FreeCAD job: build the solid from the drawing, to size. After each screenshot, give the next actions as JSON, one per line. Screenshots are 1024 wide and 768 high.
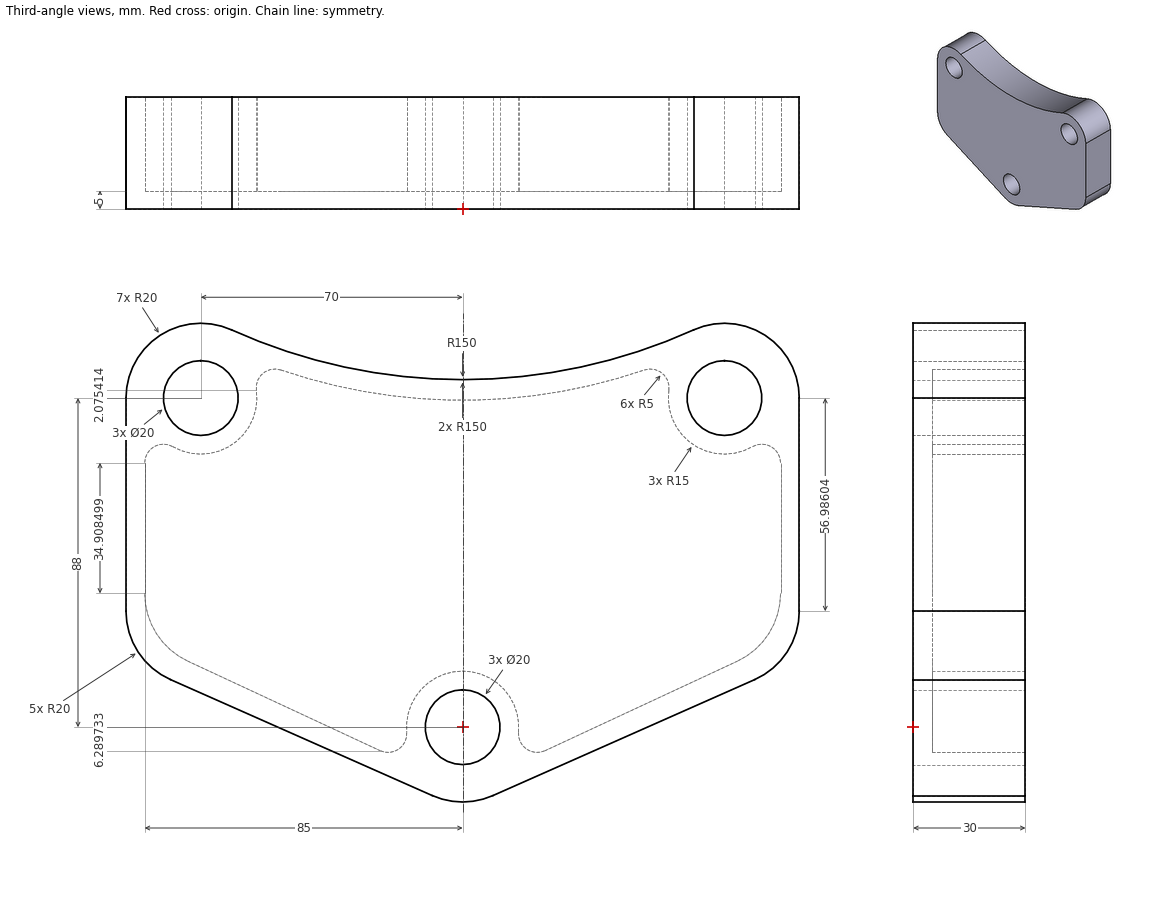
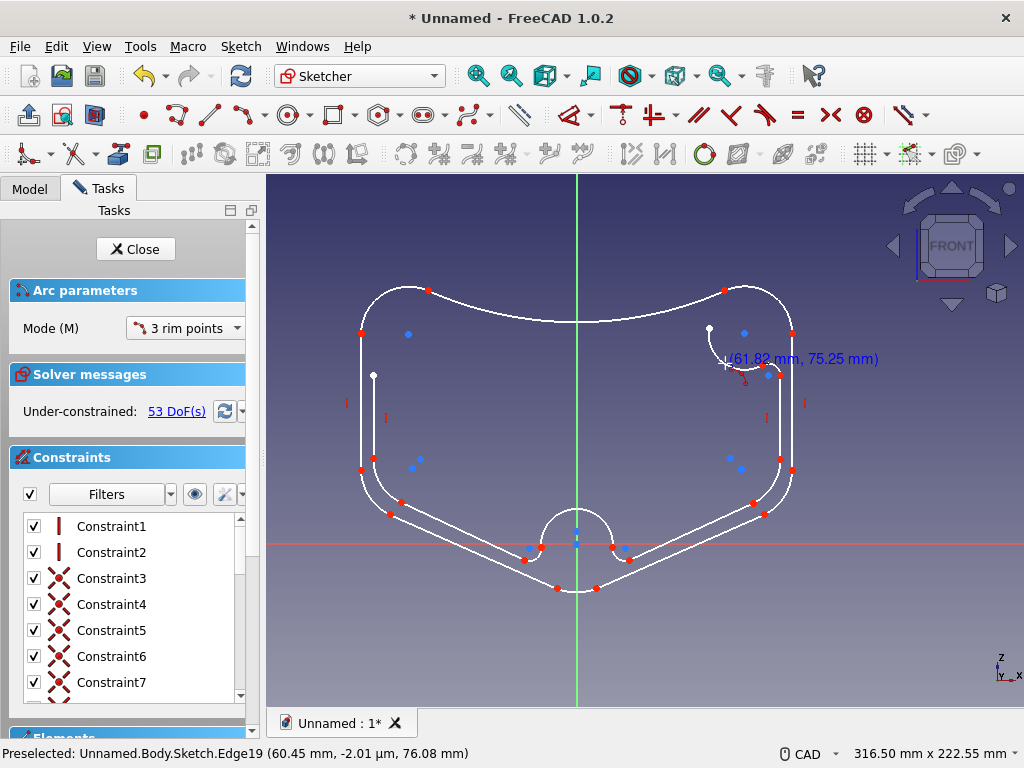
{"action": "left_click", "coordinate": [709, 329]}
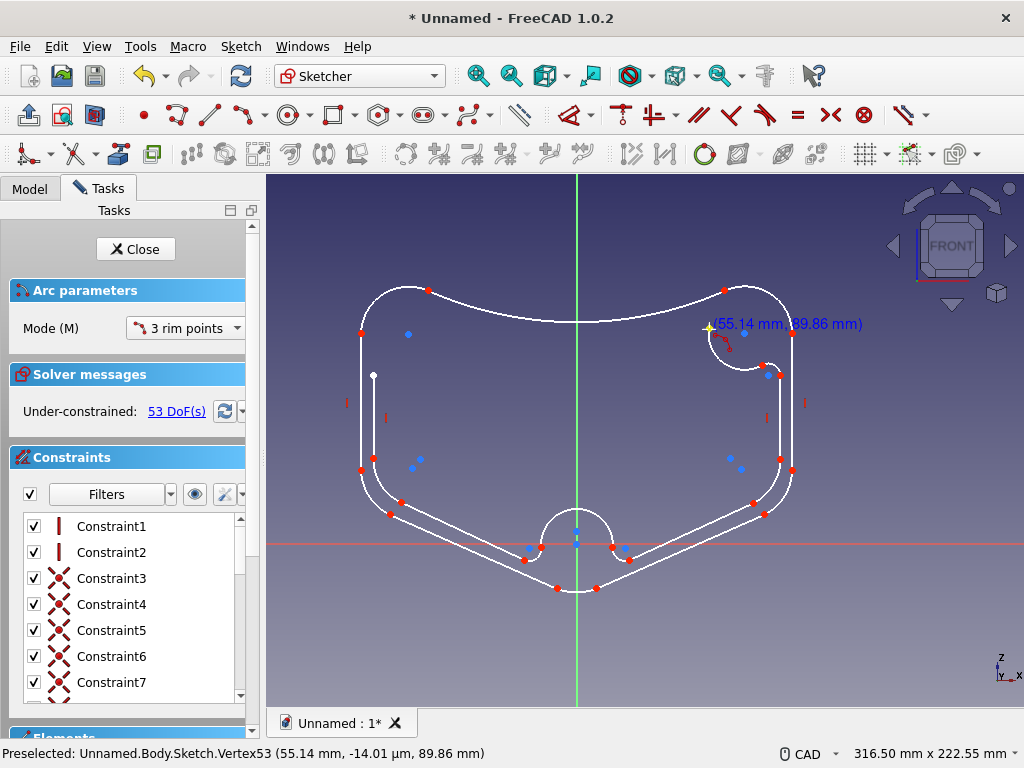
{"action": "scroll", "coordinate": [693, 316], "scroll_direction": "up", "scroll_amount": 2}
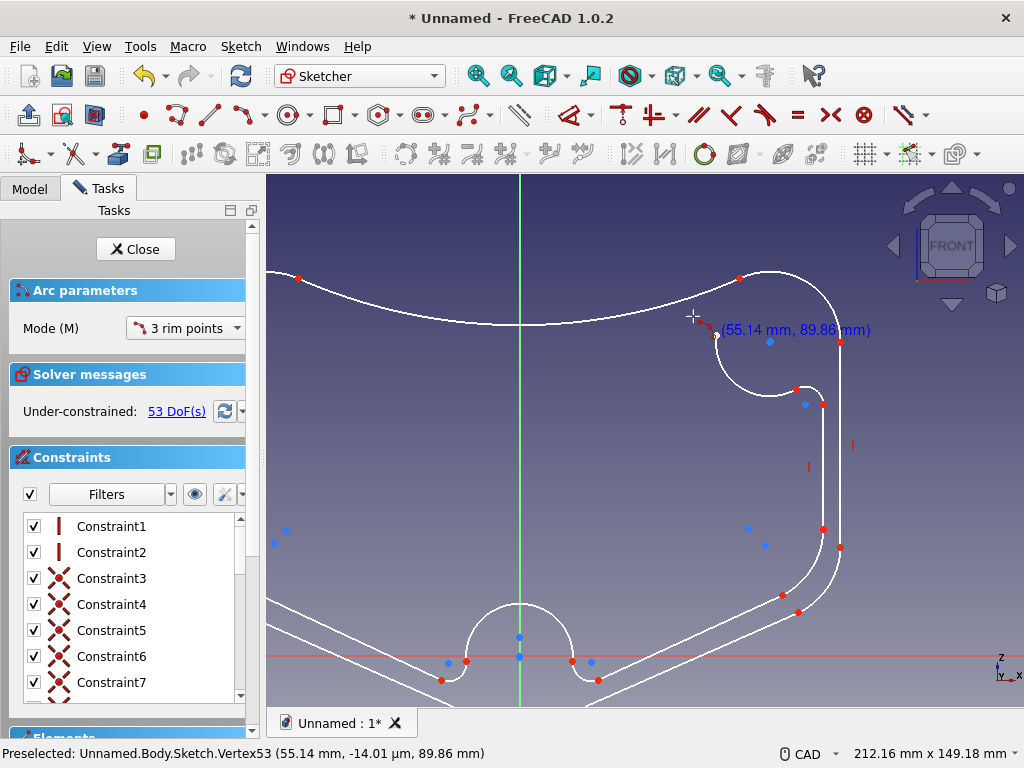
{"action": "left_click", "coordinate": [693, 315]}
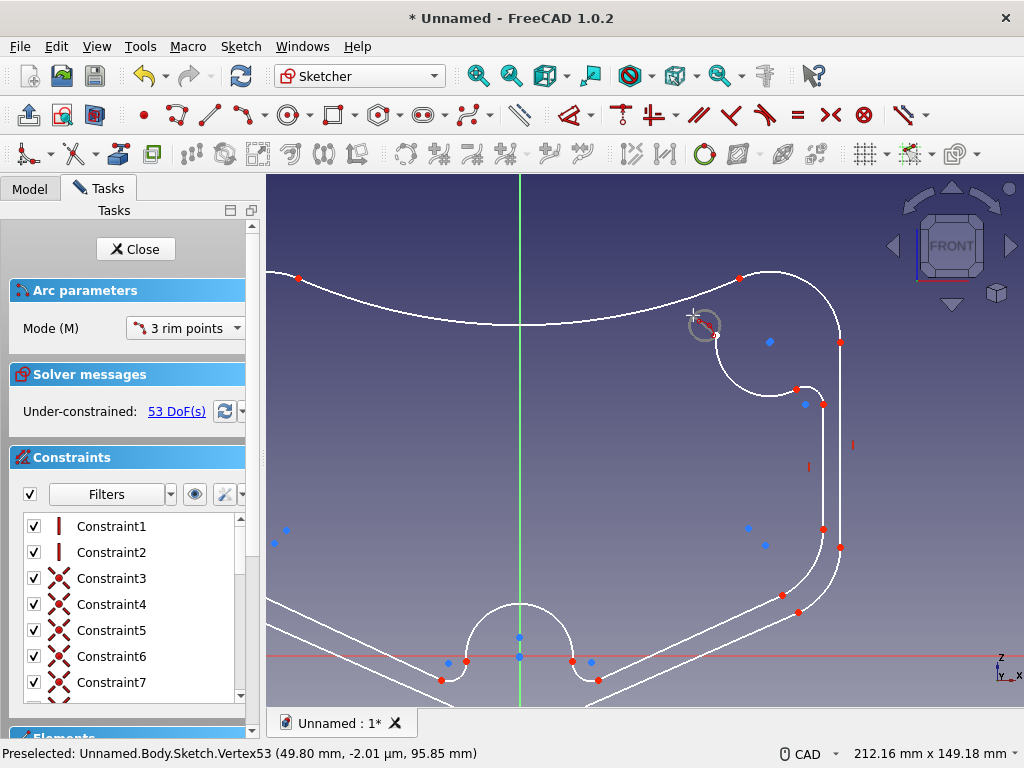
{"action": "scroll", "coordinate": [710, 318], "scroll_direction": "up", "scroll_amount": 4}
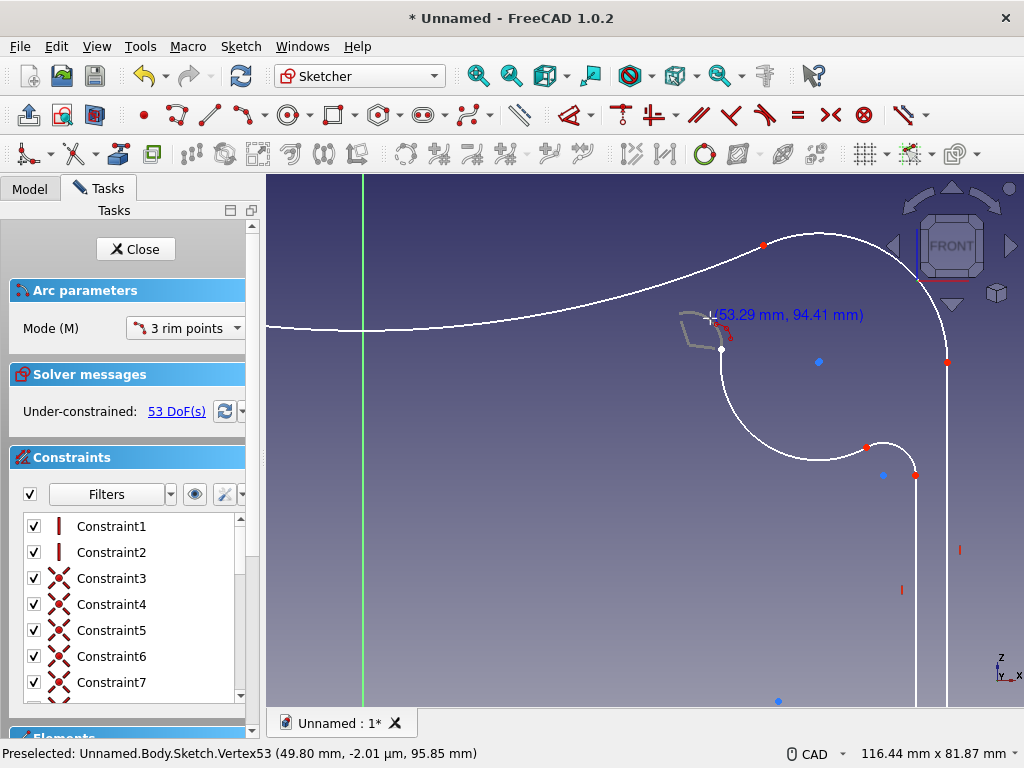
{"action": "left_click", "coordinate": [710, 318]}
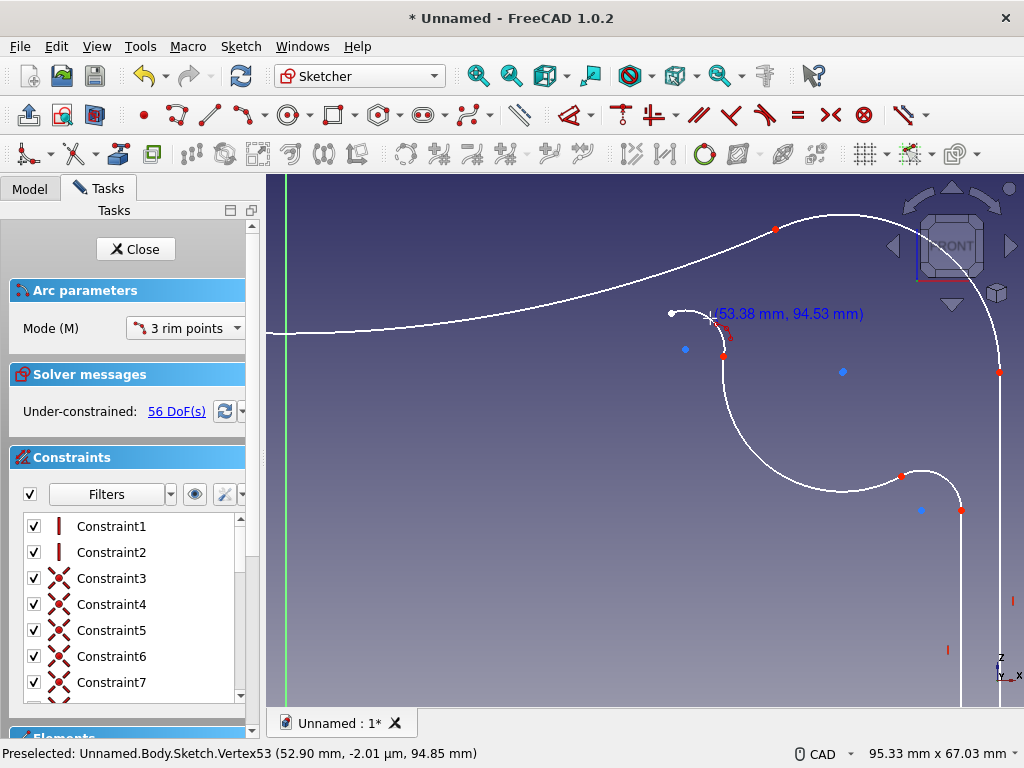
{"action": "left_click", "coordinate": [671, 313]}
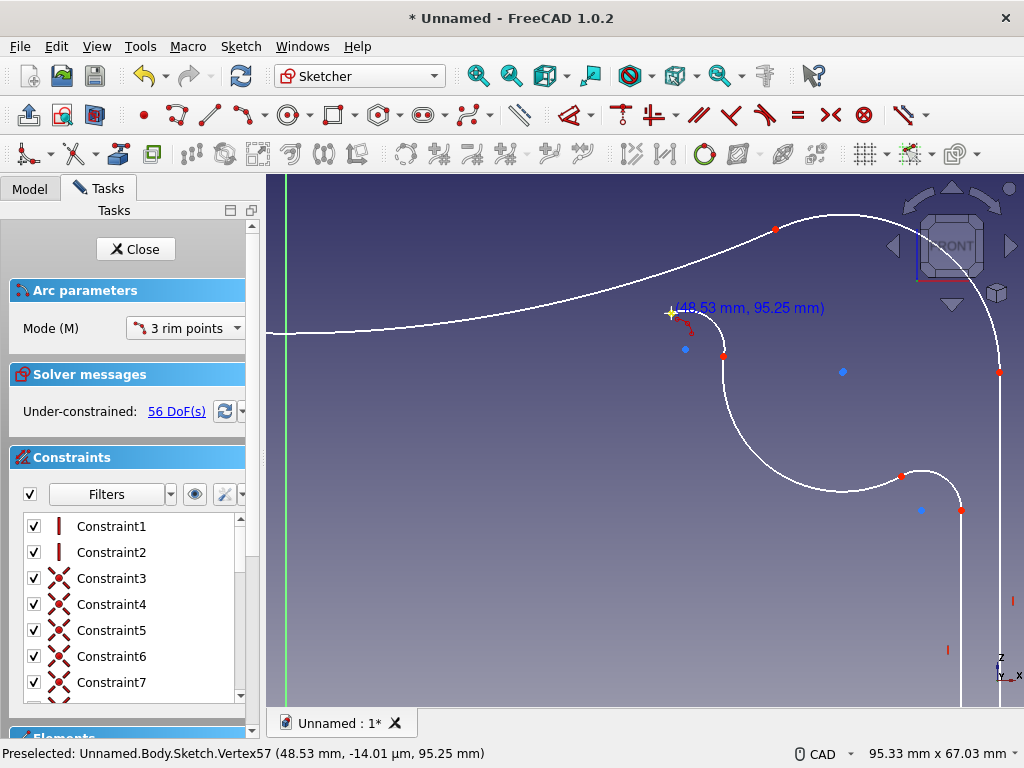
{"action": "scroll", "coordinate": [702, 317], "scroll_direction": "down", "scroll_amount": 6}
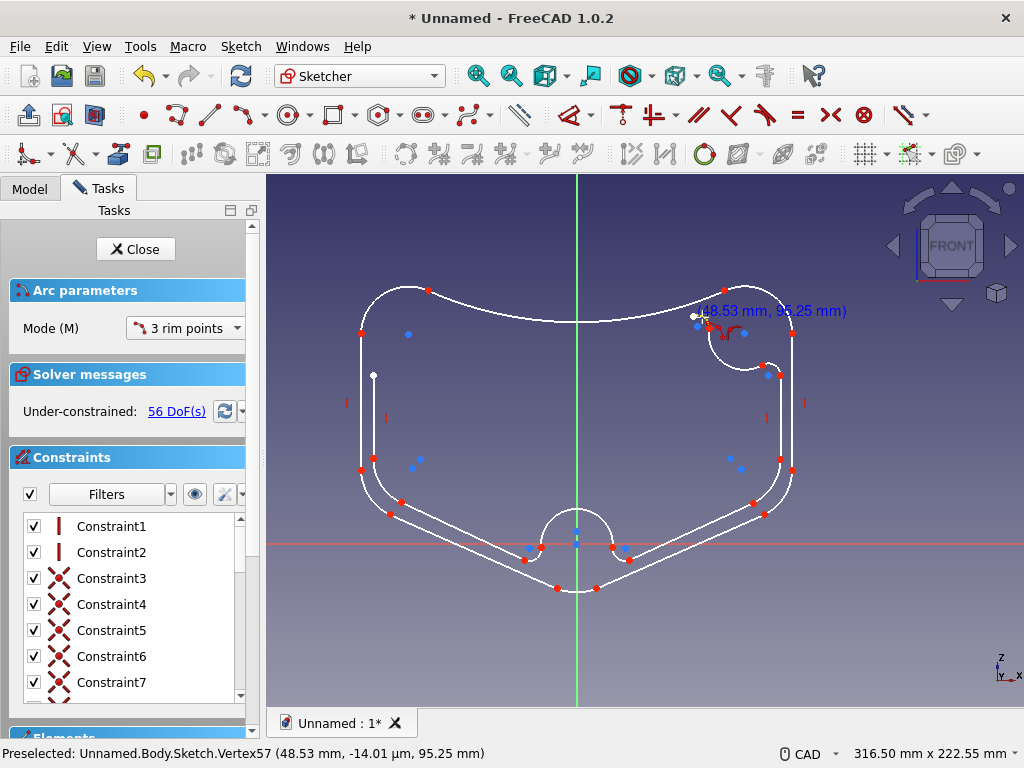
{"action": "scroll", "coordinate": [461, 315], "scroll_direction": "up", "scroll_amount": 2}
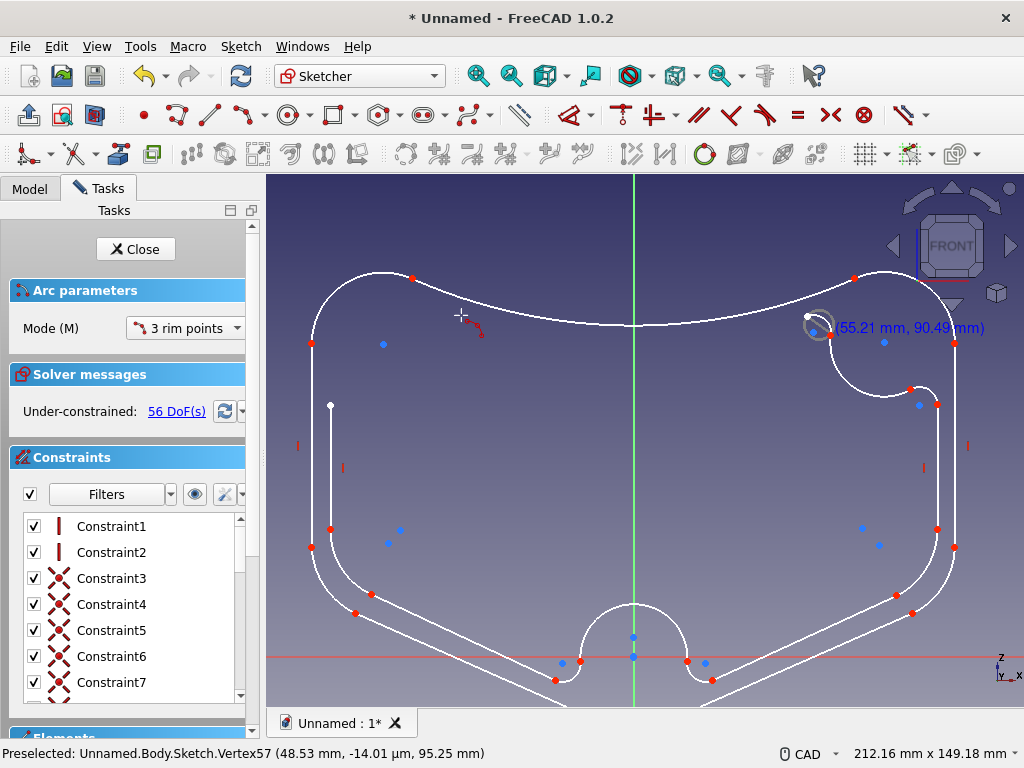
{"action": "left_click", "coordinate": [460, 316]}
{"action": "left_click", "coordinate": [599, 343]}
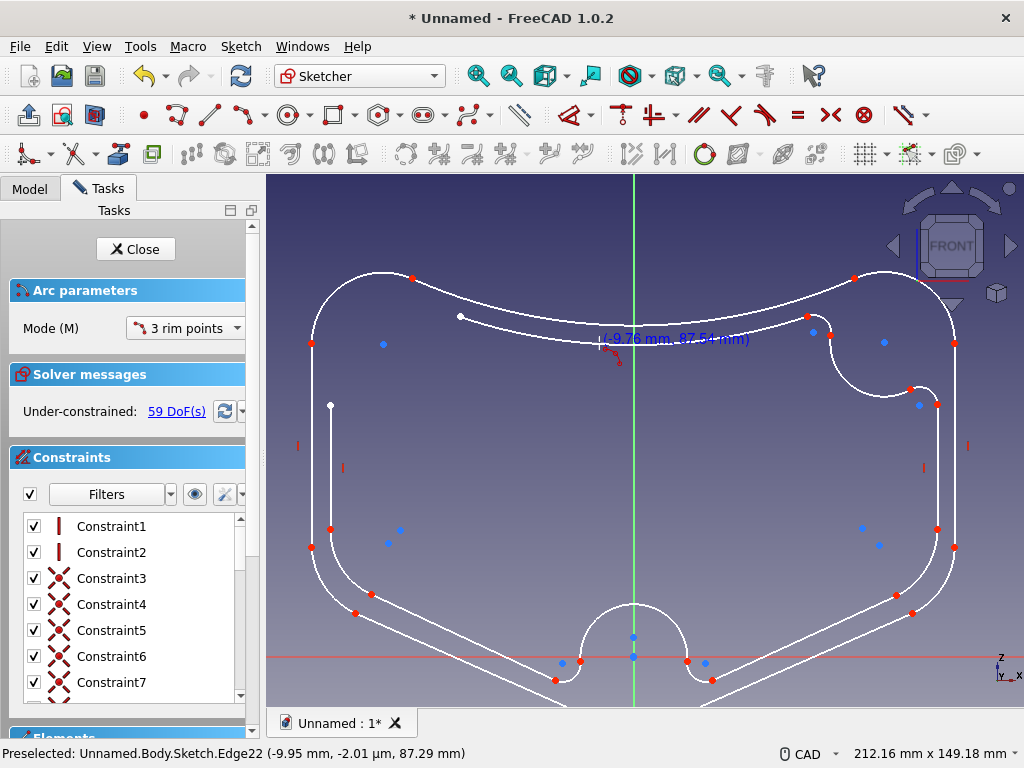
{"action": "left_click", "coordinate": [460, 317]}
{"action": "left_click", "coordinate": [437, 335]}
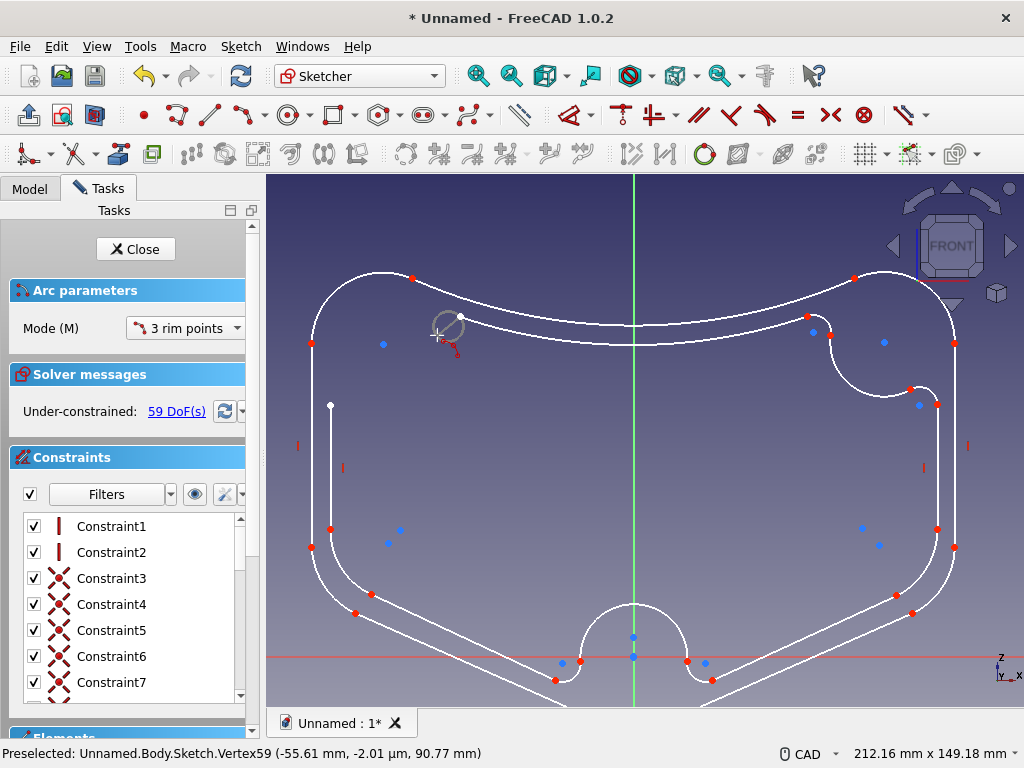
{"action": "scroll", "coordinate": [443, 319], "scroll_direction": "up", "scroll_amount": 4}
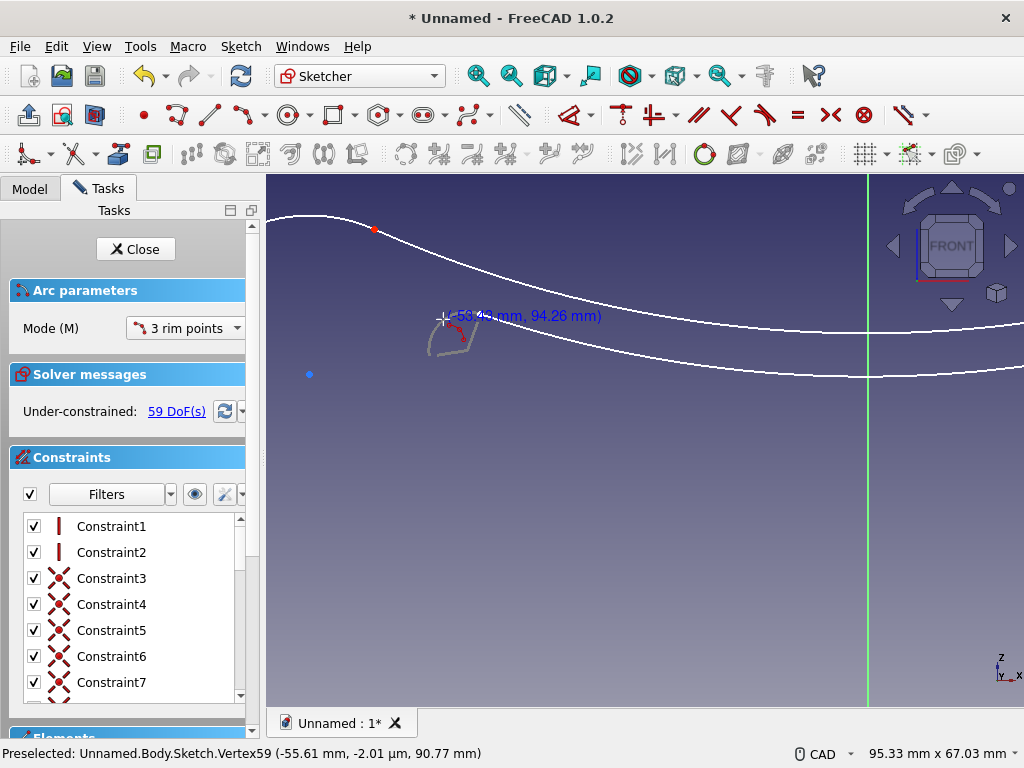
{"action": "left_click", "coordinate": [443, 318]}